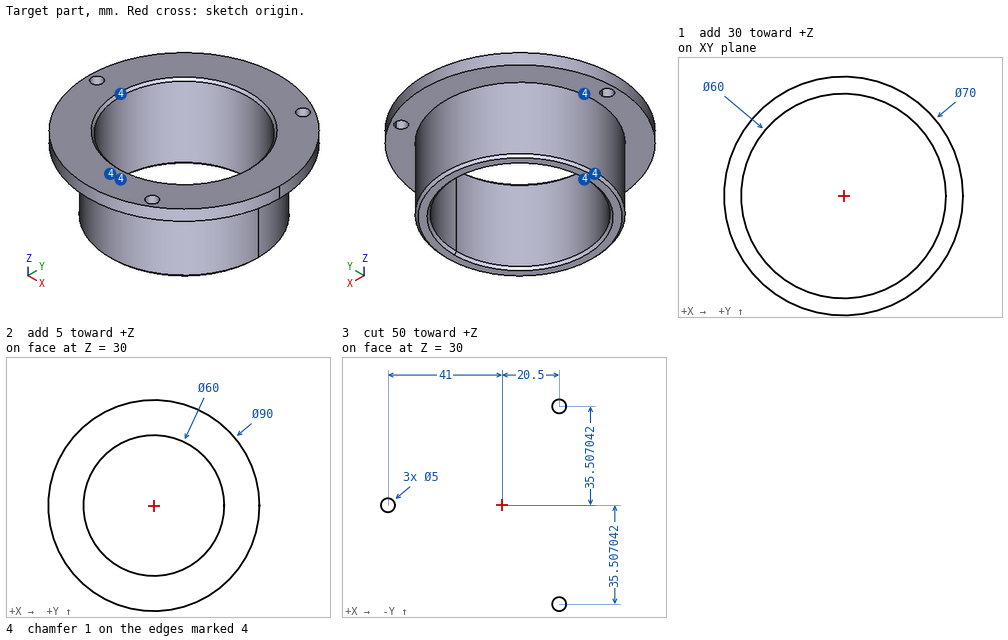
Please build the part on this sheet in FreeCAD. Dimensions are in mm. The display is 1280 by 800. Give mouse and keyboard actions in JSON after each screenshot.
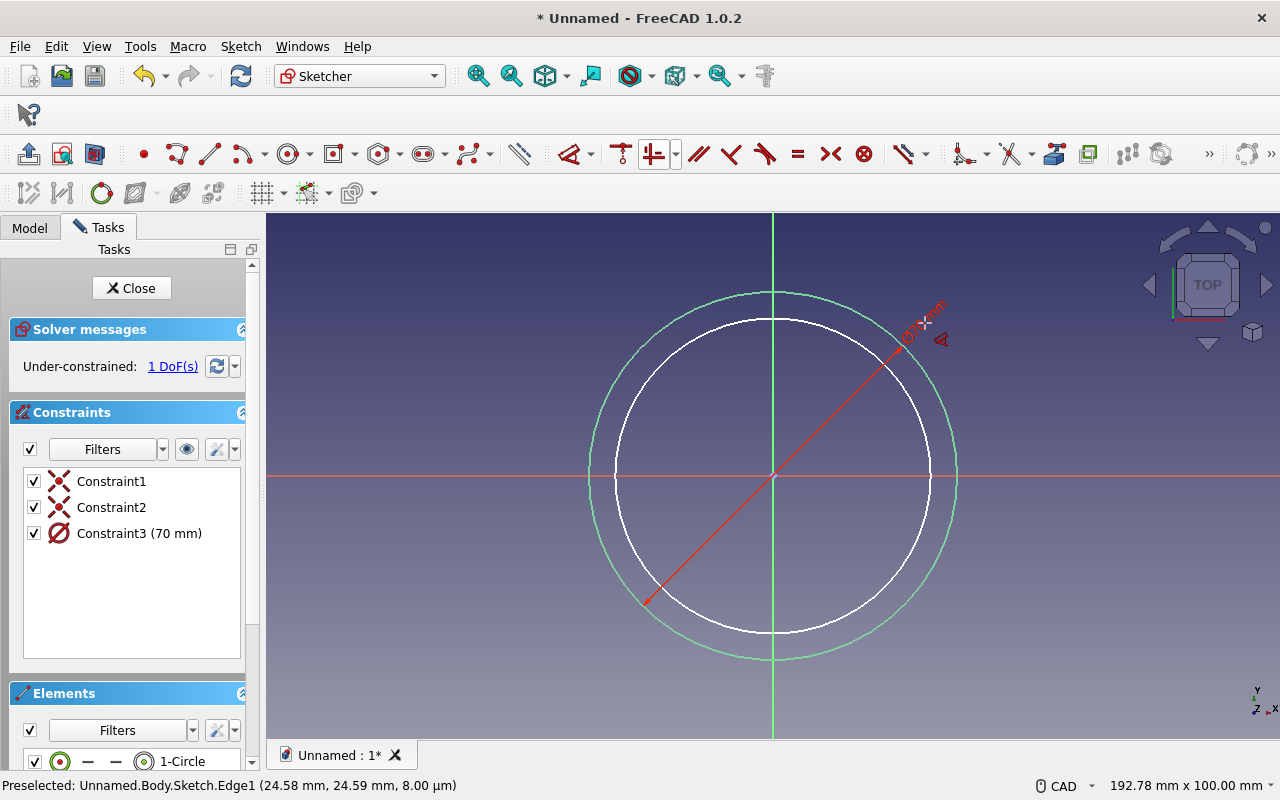
{"action": "left_click", "coordinate": [884, 364]}
{"action": "left_click", "coordinate": [977, 415]}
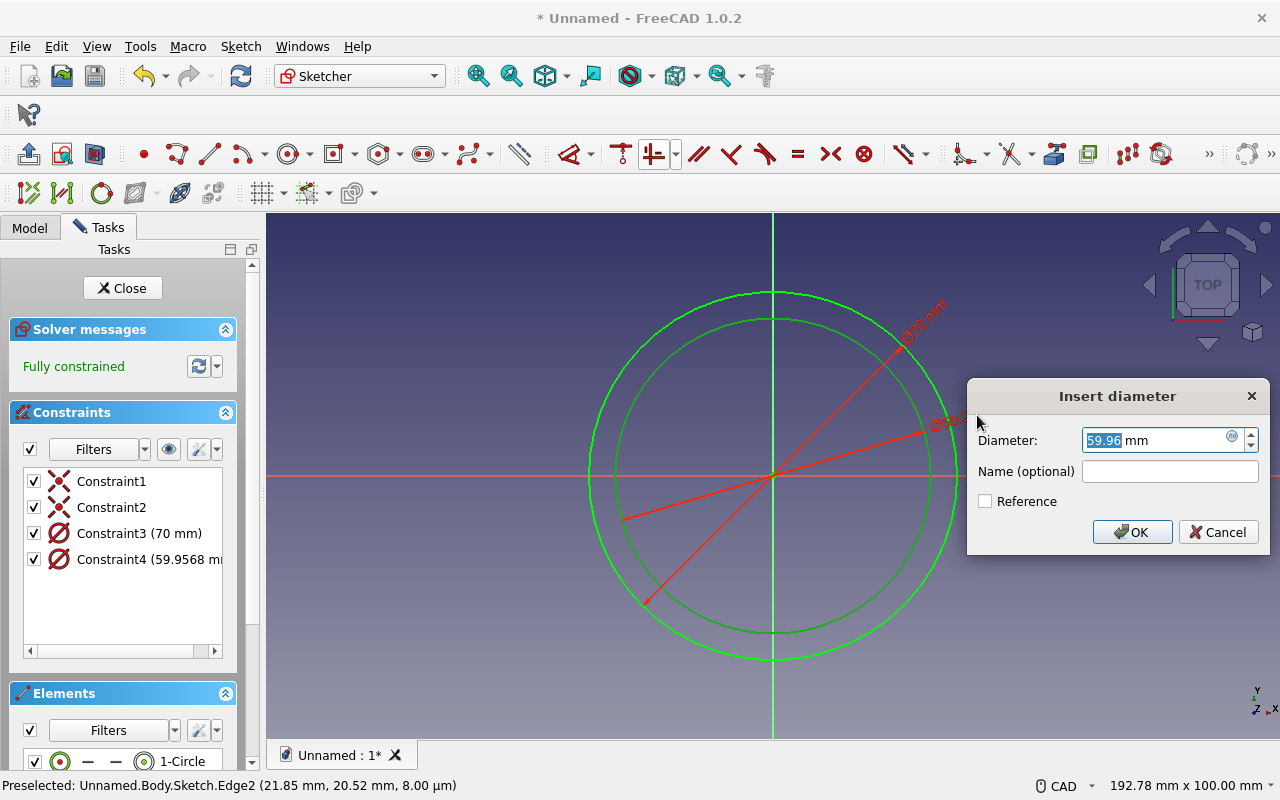
{"action": "type", "text": "60"}
{"action": "key", "text": "Return"}
{"action": "key", "text": "Escape"}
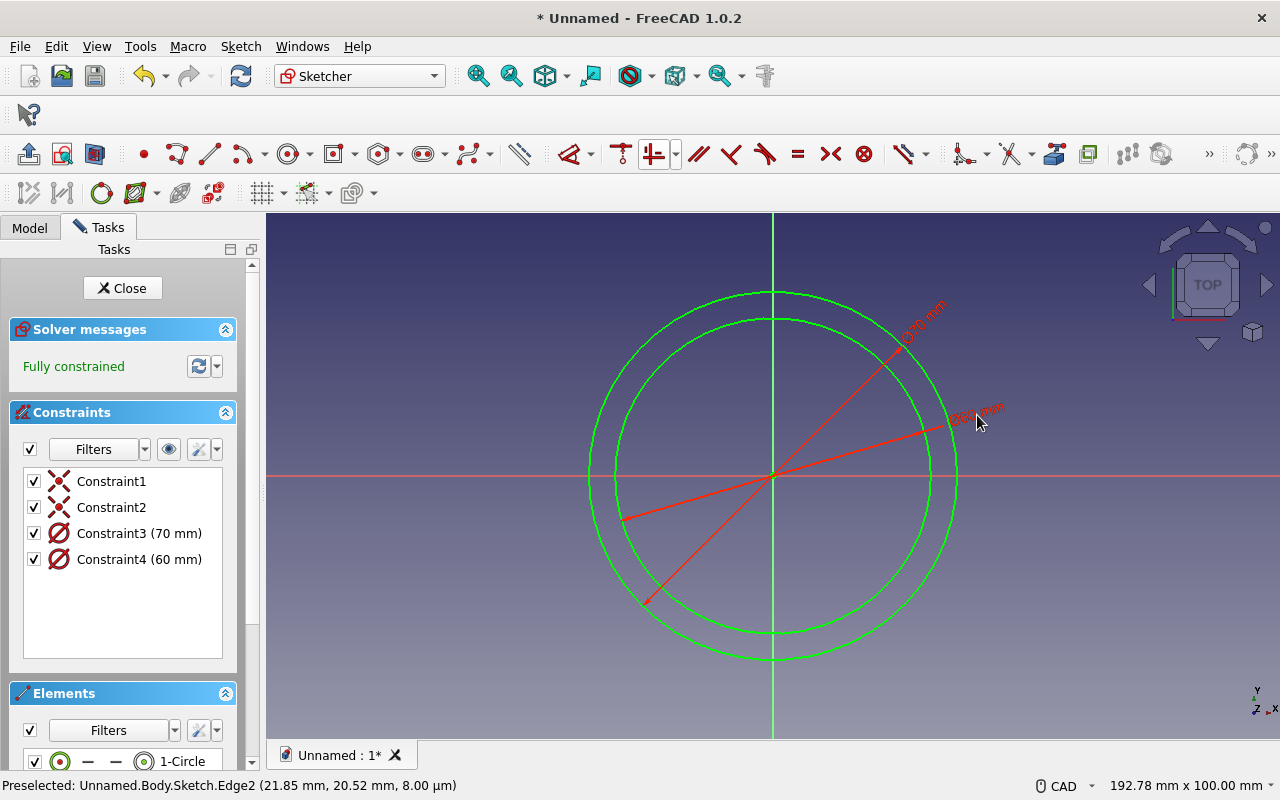
{"action": "left_click", "coordinate": [123, 288]}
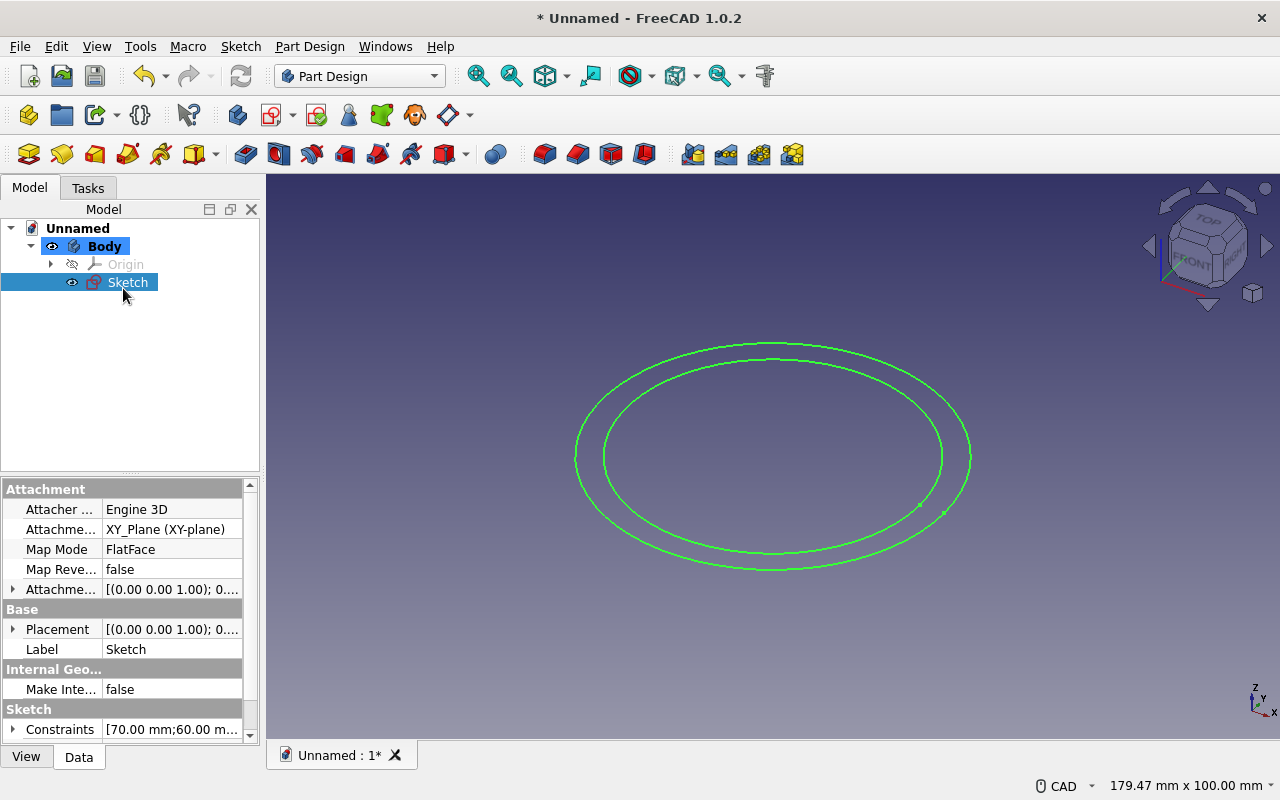
{"action": "left_click", "coordinate": [29, 154]}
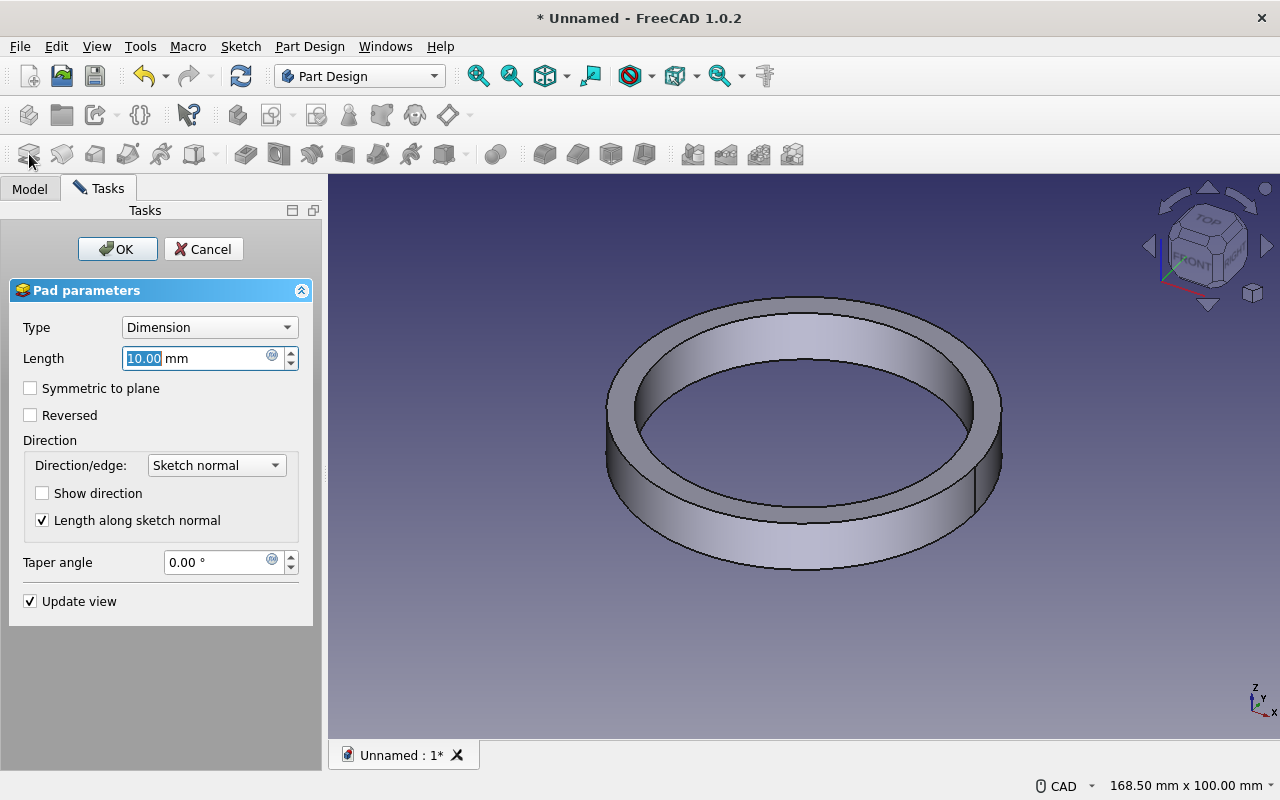
{"action": "type", "text": "30"}
{"action": "key", "text": "Tab"}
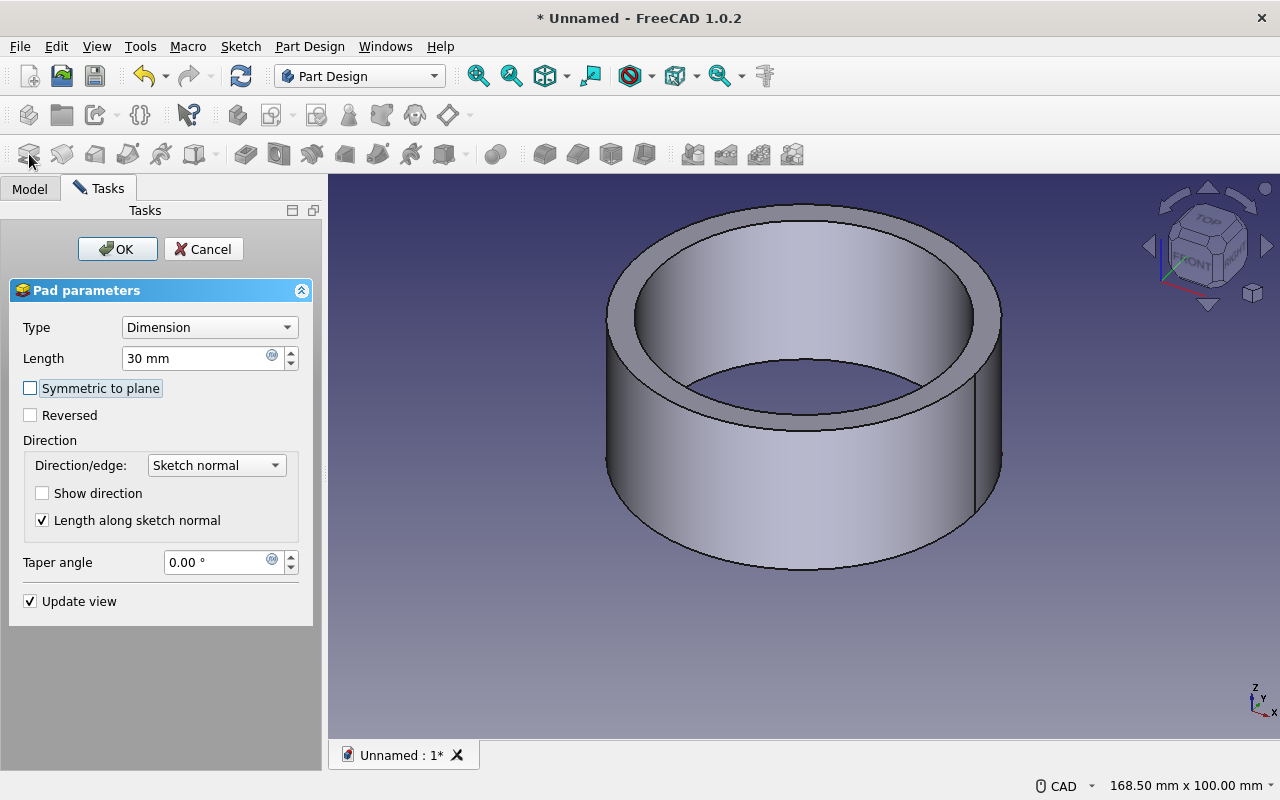
{"action": "left_click", "coordinate": [118, 249]}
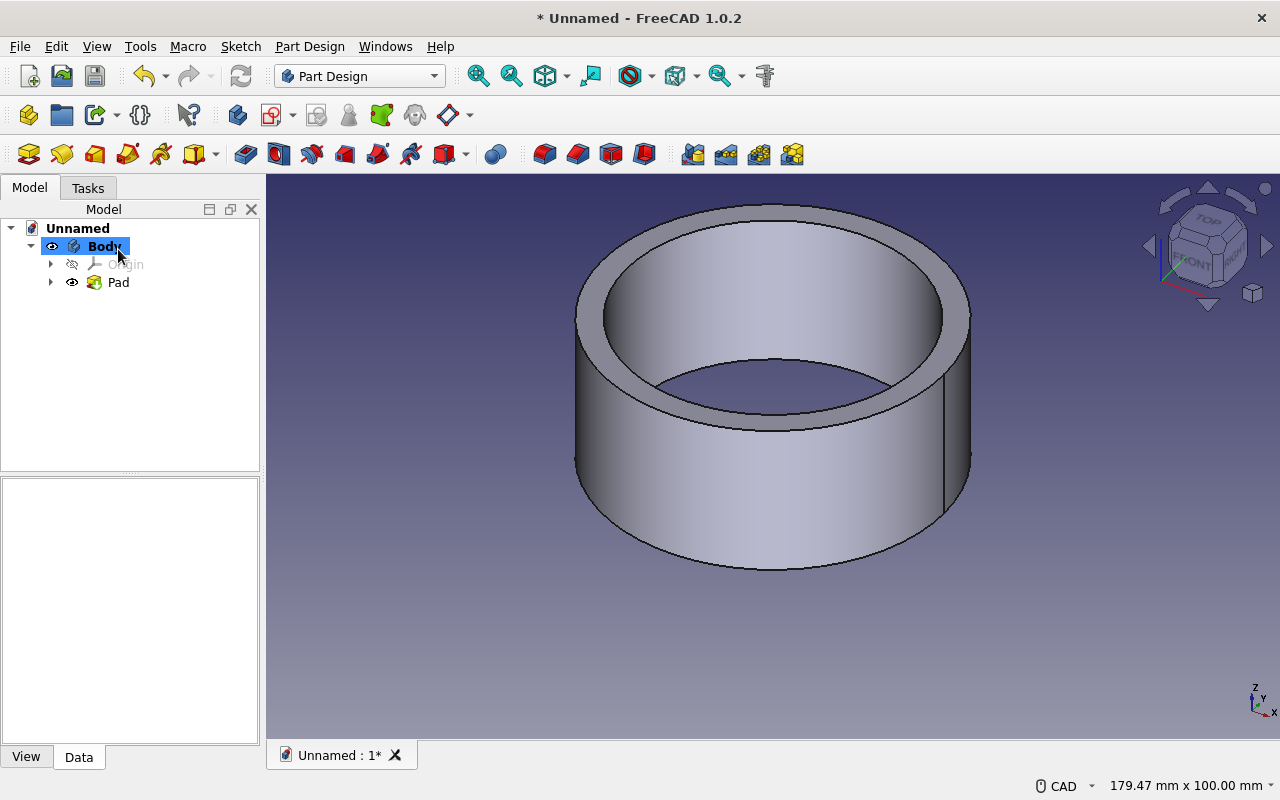
{"action": "key", "text": "v f"}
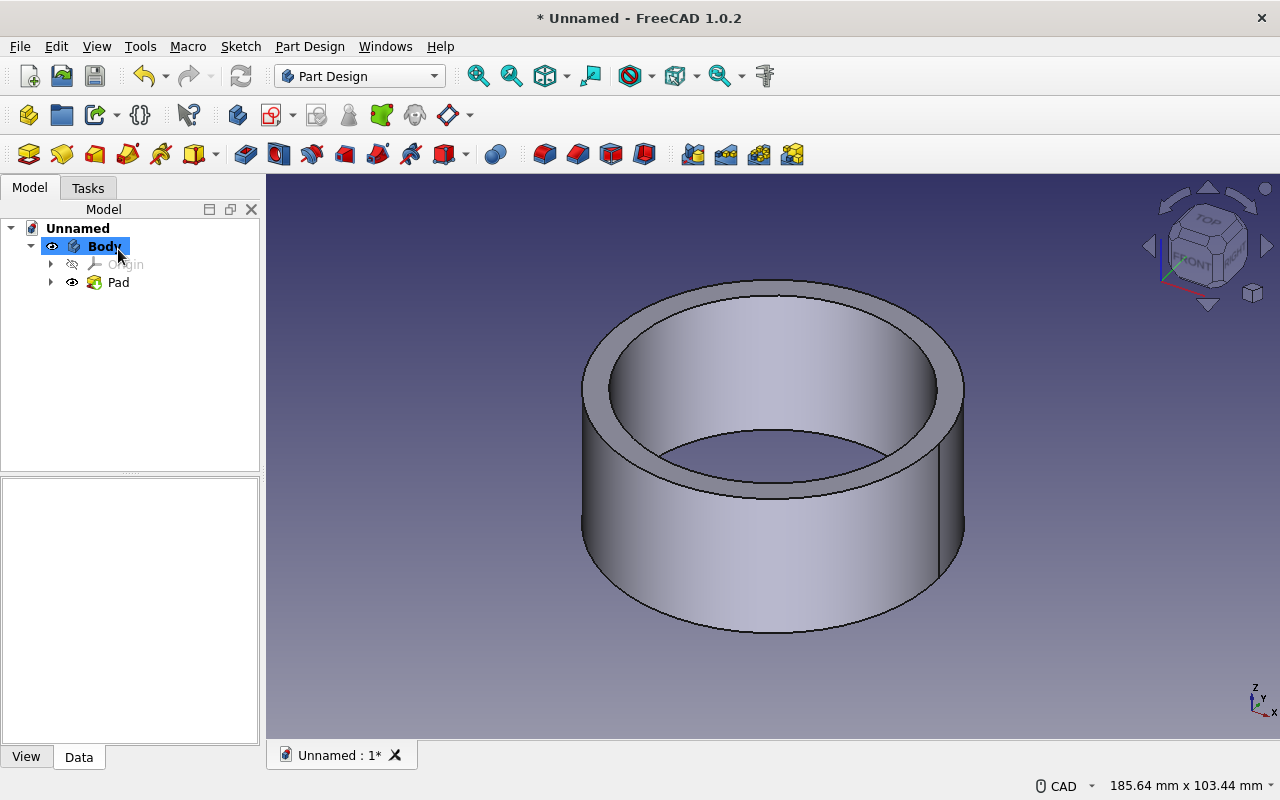
{"action": "left_click", "coordinate": [942, 408]}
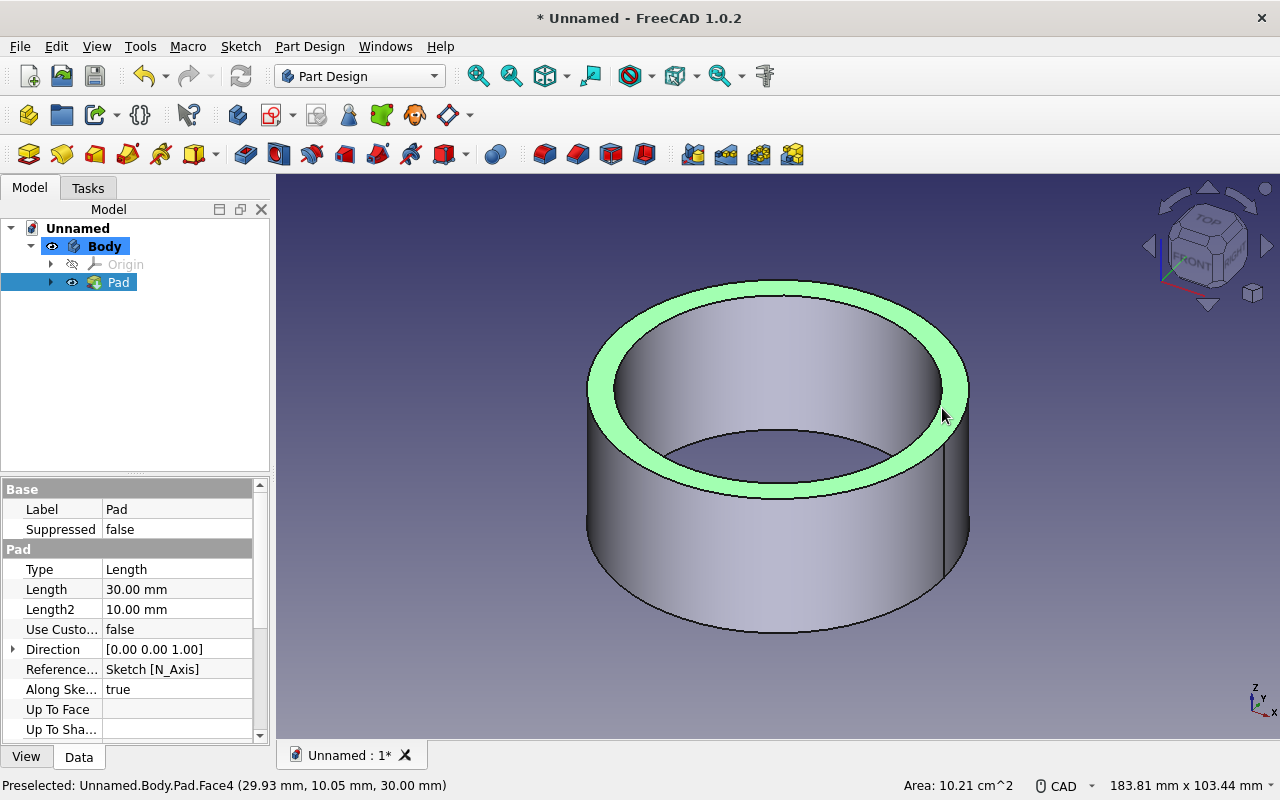
{"action": "left_click", "coordinate": [270, 116]}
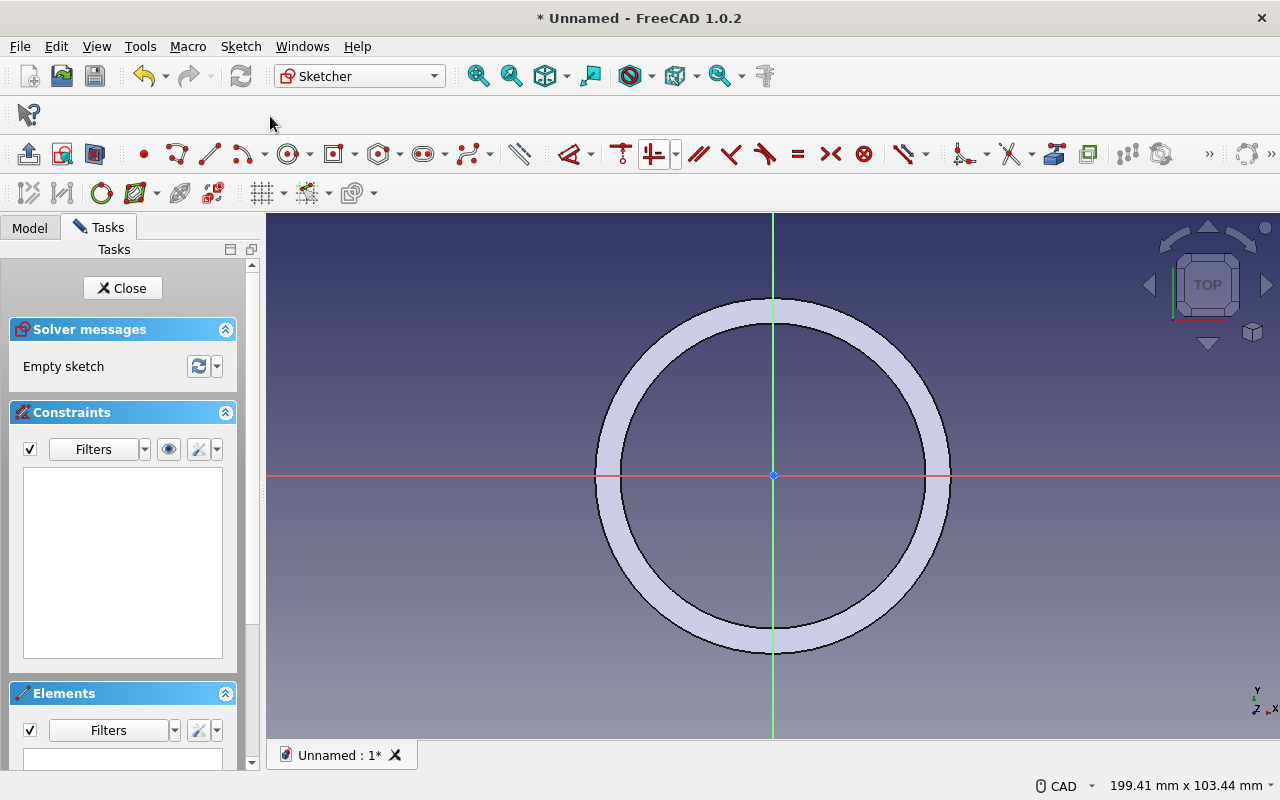
{"action": "scroll", "coordinate": [565, 476], "scroll_direction": "down", "scroll_amount": 2}